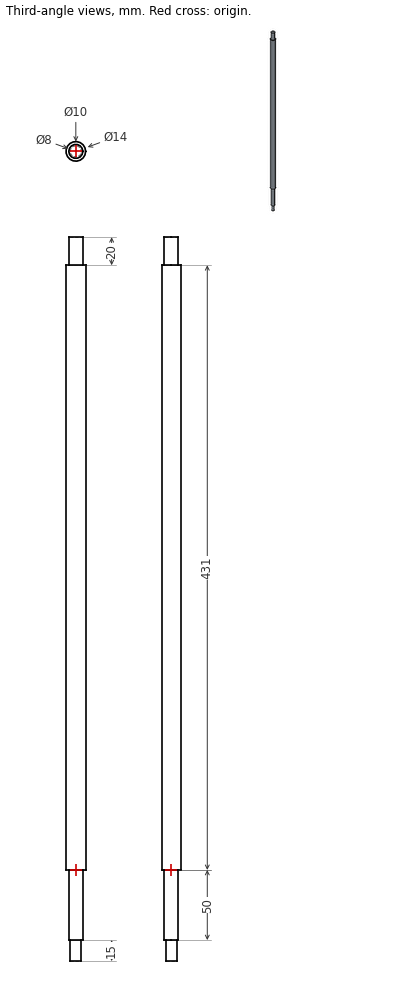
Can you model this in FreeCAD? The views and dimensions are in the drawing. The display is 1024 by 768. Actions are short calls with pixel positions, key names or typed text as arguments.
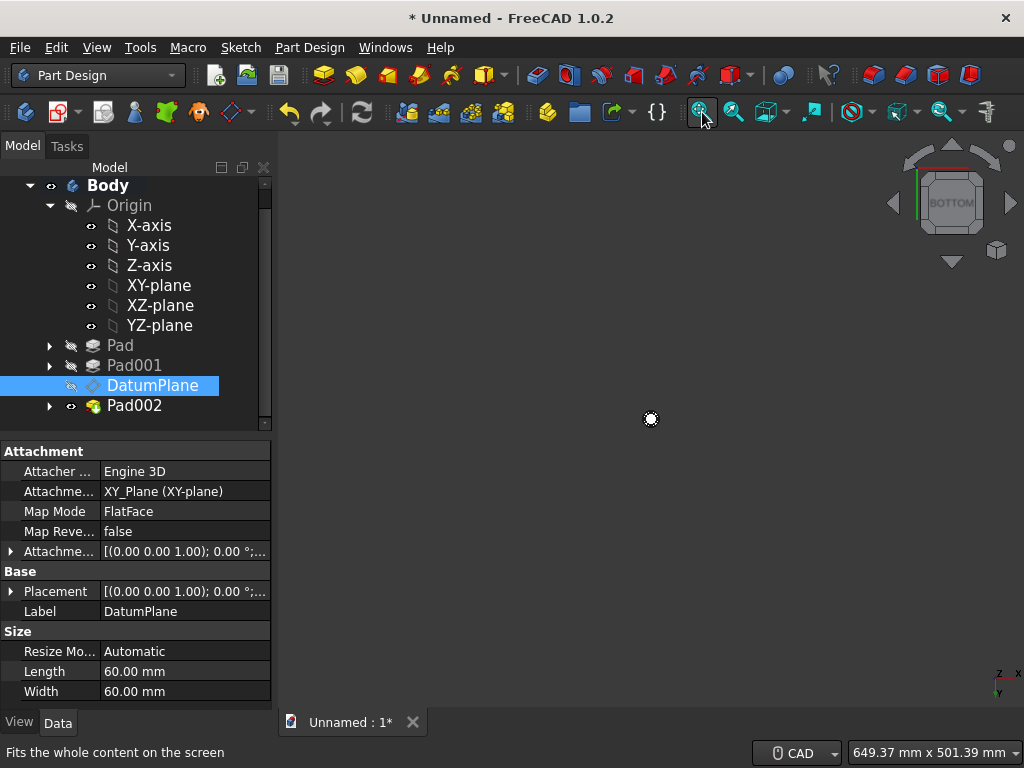
click(702, 112)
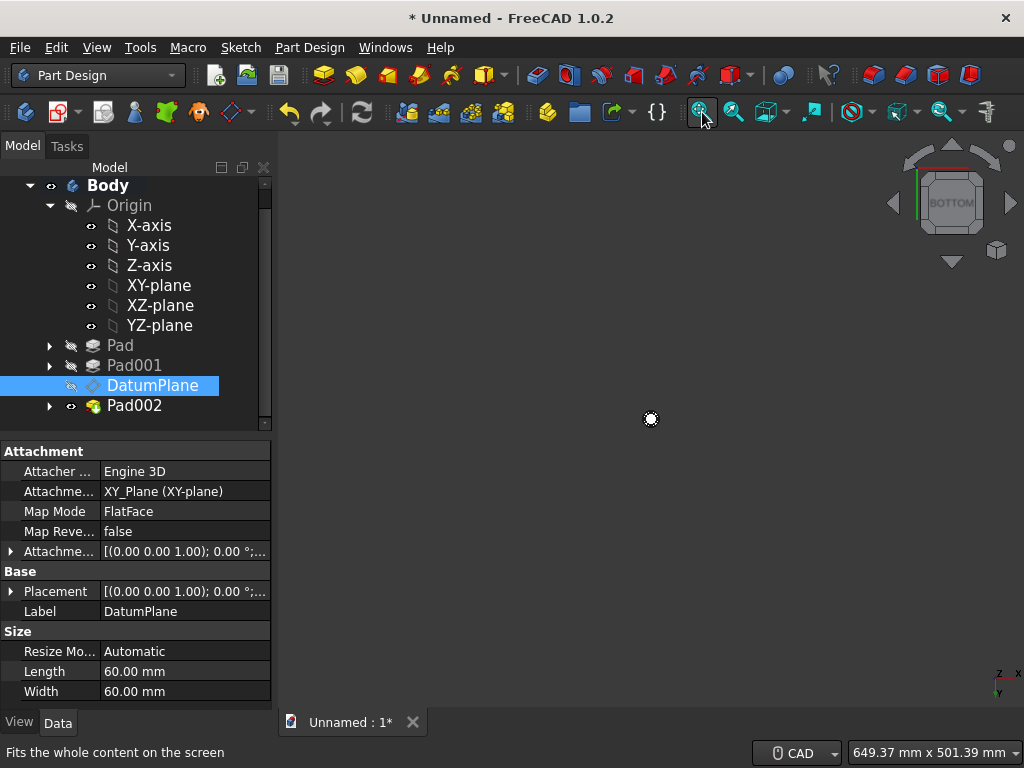
scroll(651, 418, up, 4)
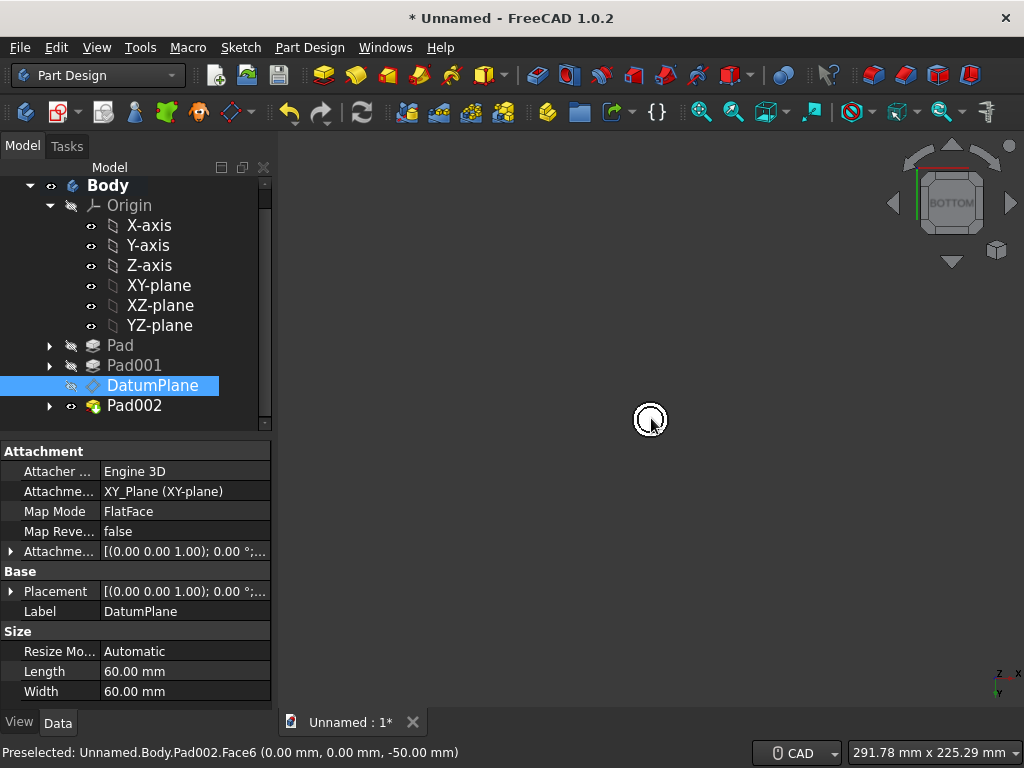
click(650, 419)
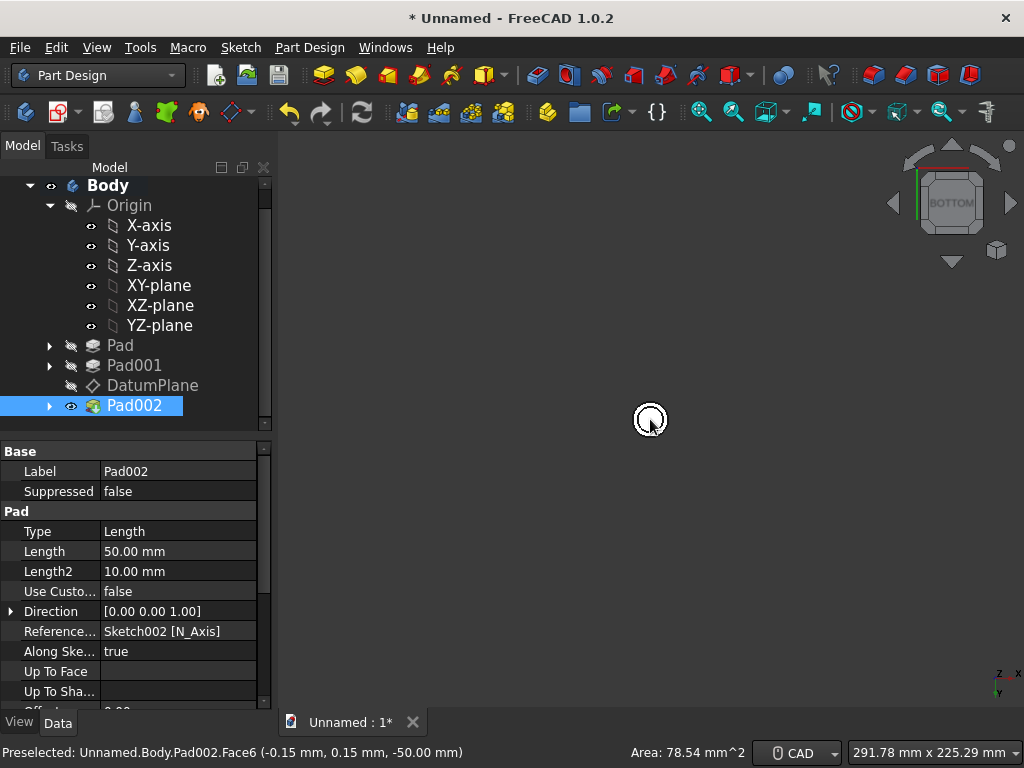
click(58, 112)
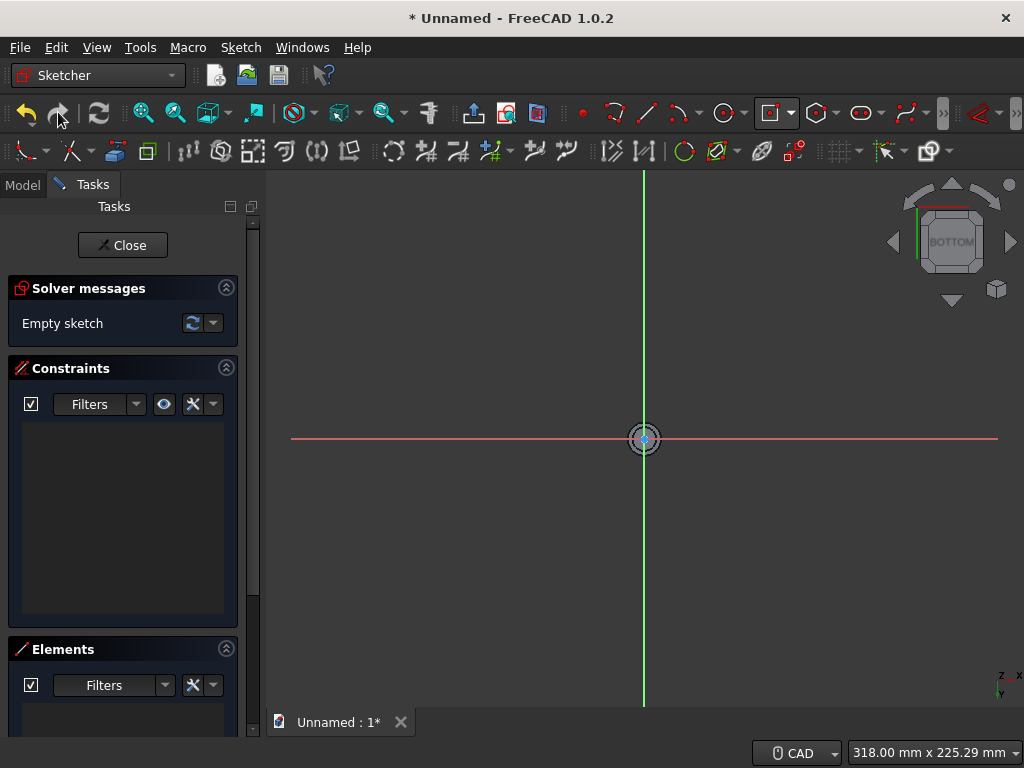
scroll(649, 439, up, 14)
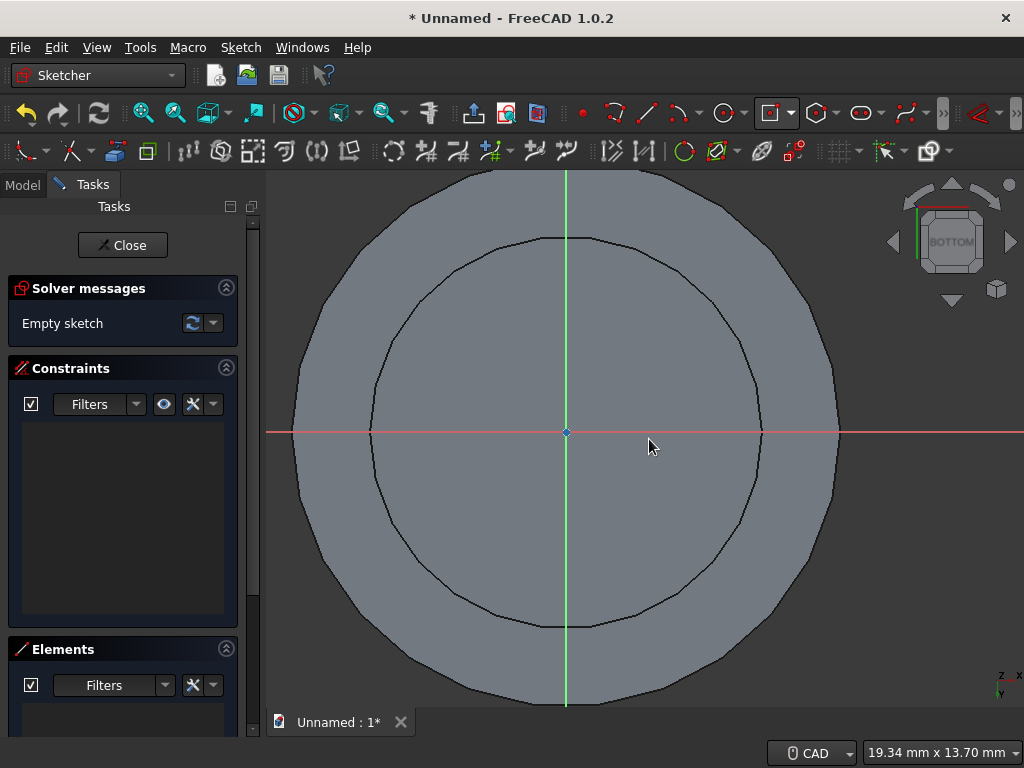
click(724, 114)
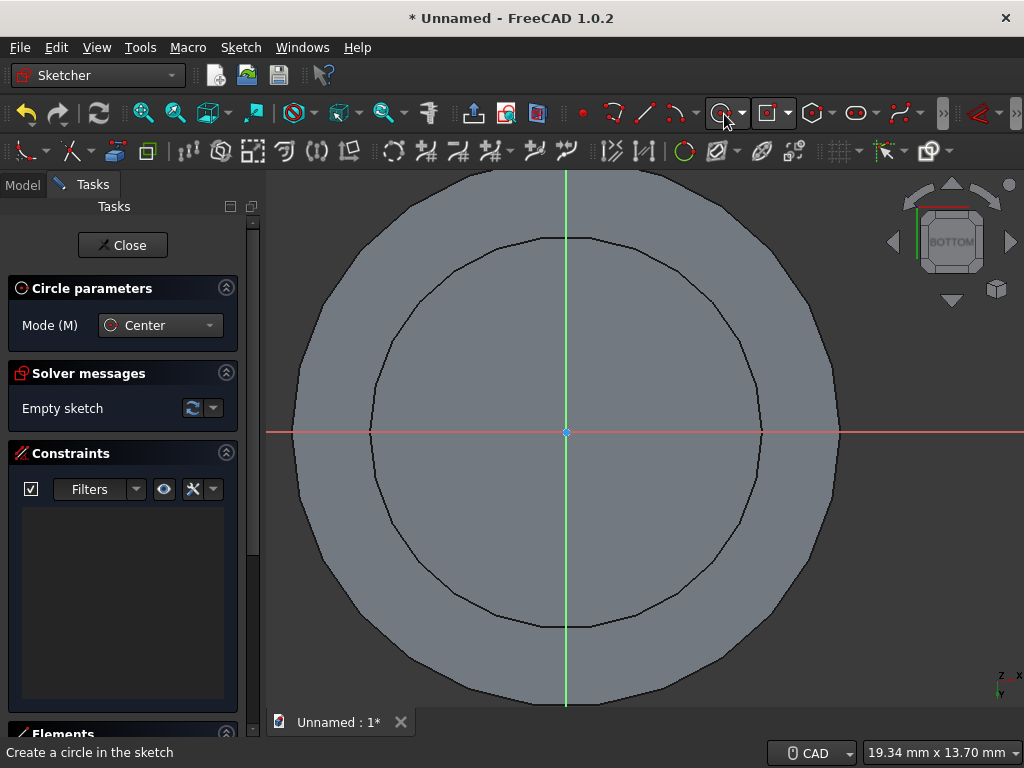
click(566, 432)
move(677, 322)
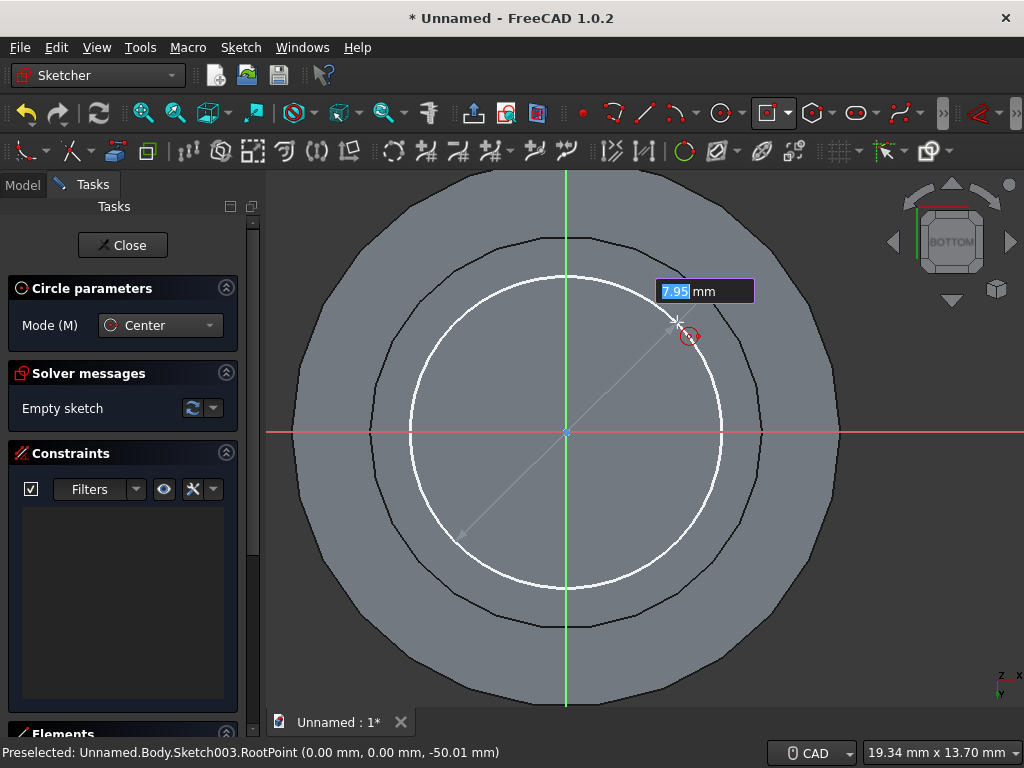
text(8)
key(Return)
key(Escape)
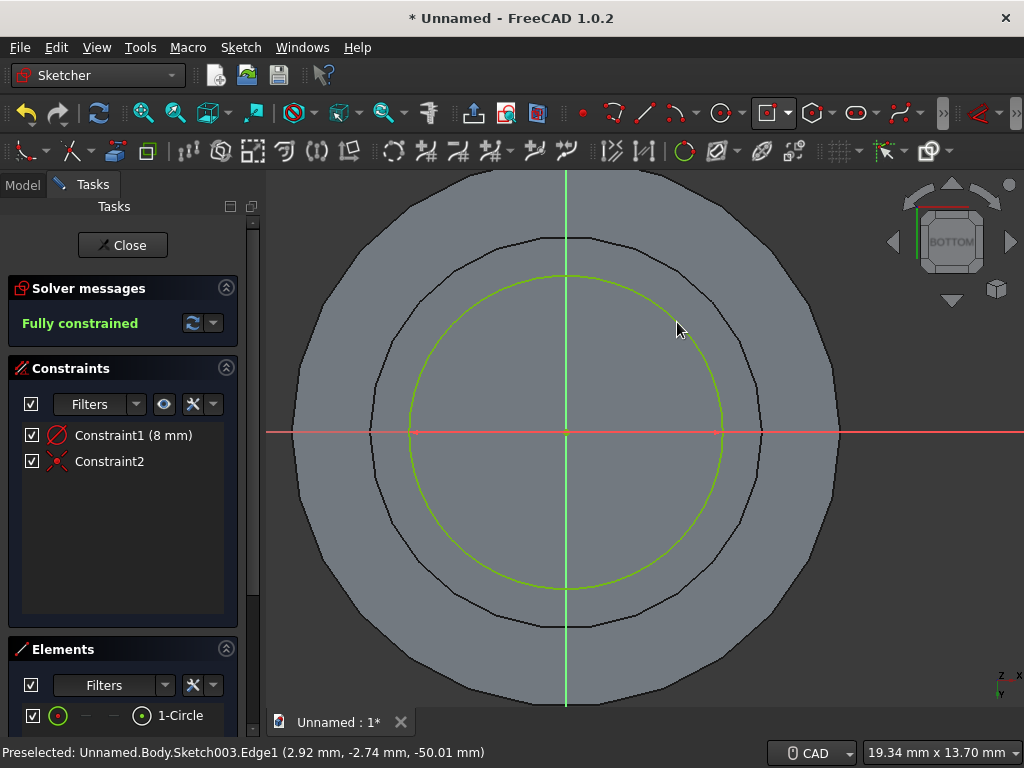
click(123, 245)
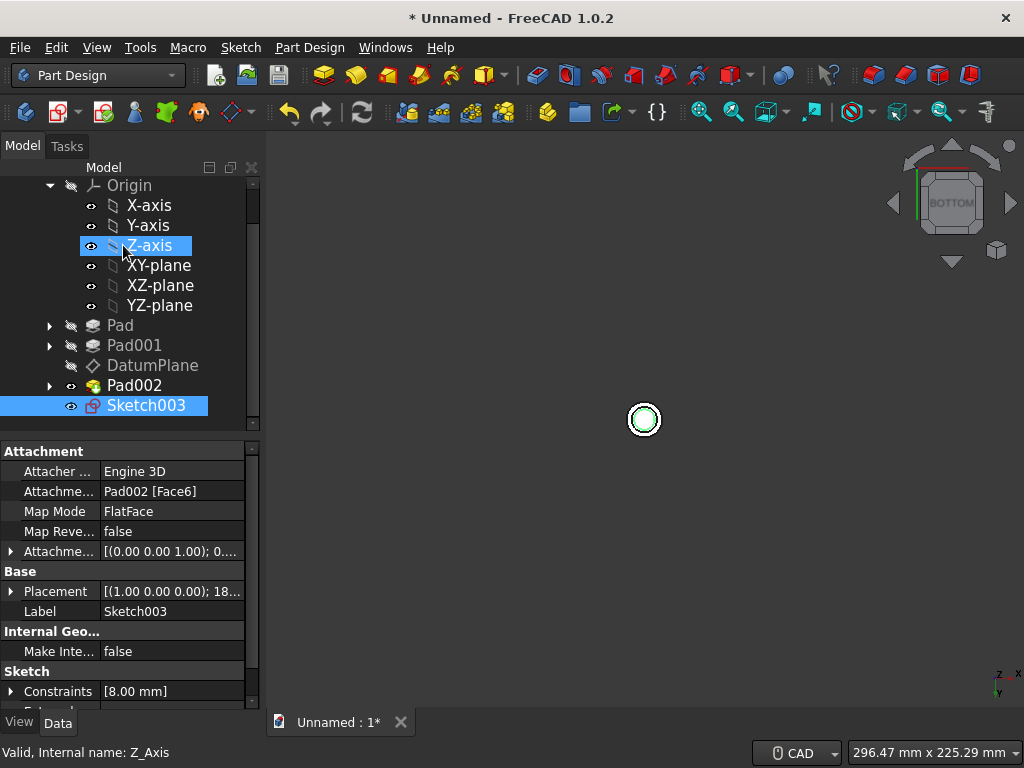
click(324, 76)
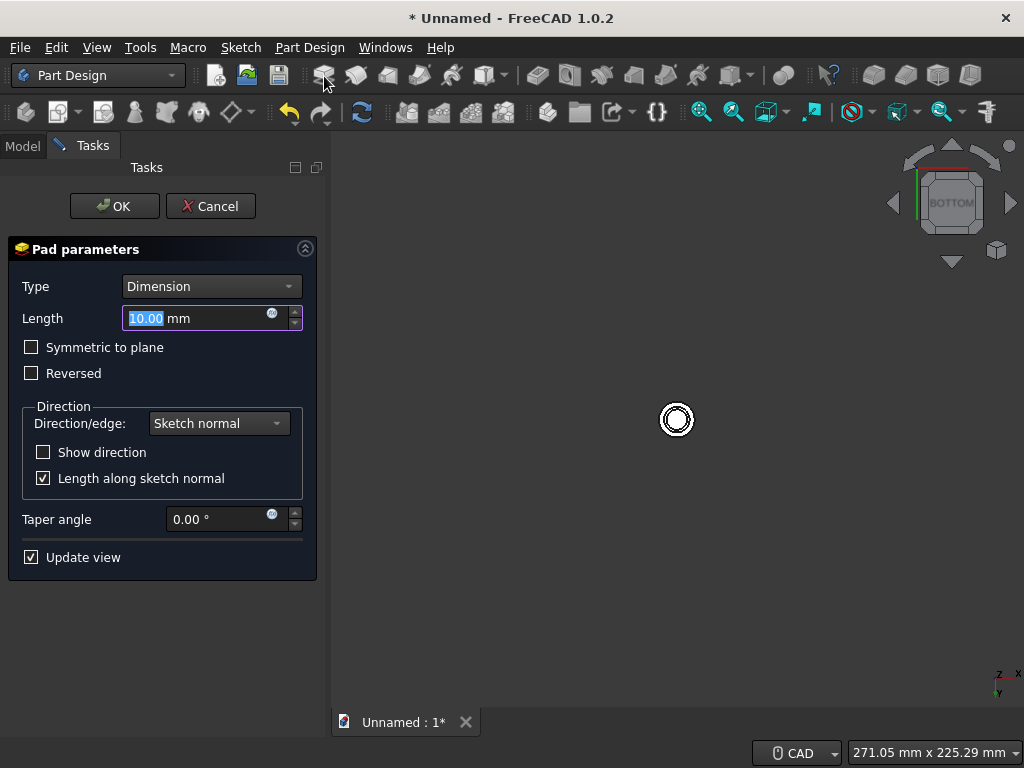
text(15)
key(Tab)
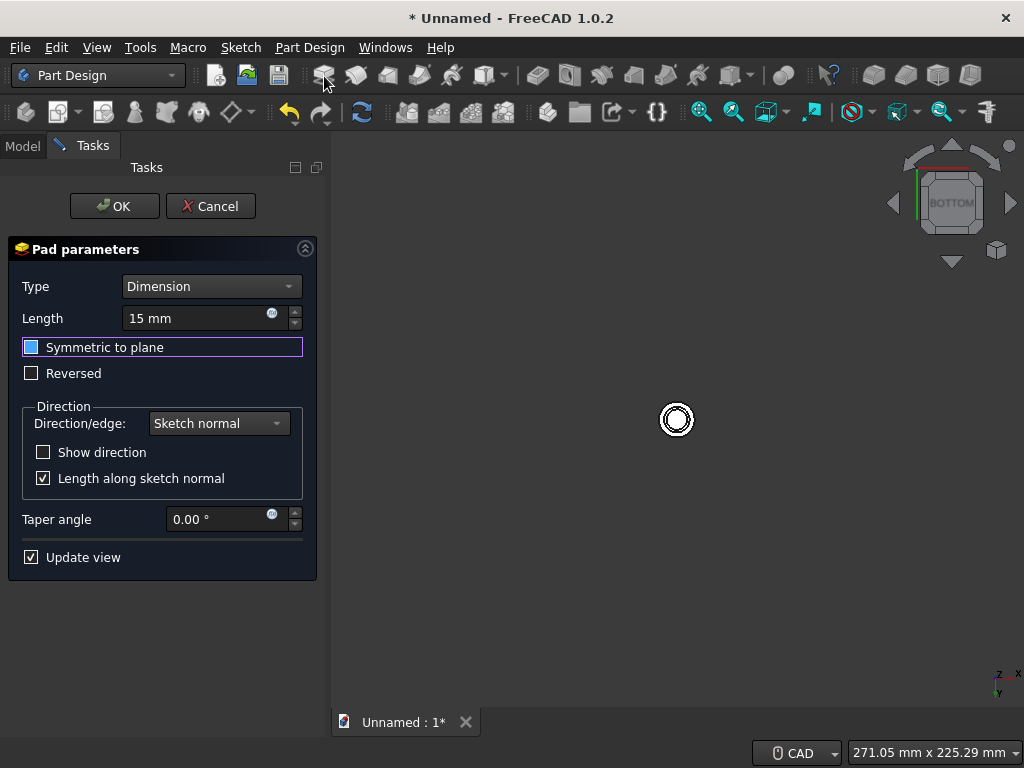
click(115, 206)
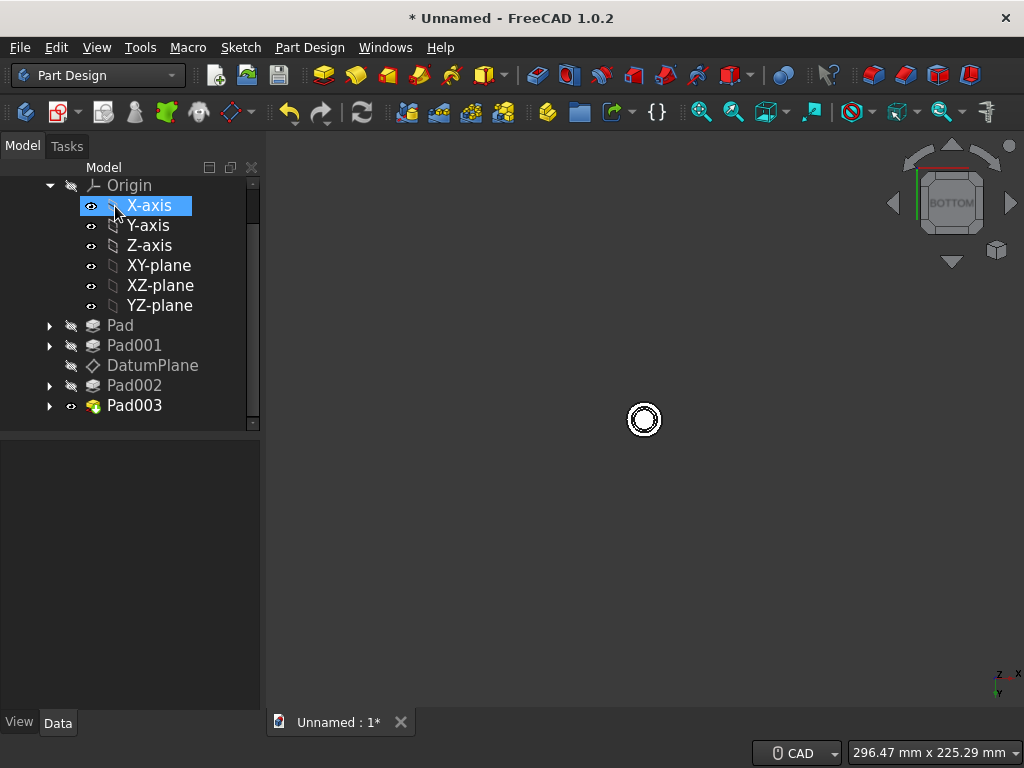
key(0)